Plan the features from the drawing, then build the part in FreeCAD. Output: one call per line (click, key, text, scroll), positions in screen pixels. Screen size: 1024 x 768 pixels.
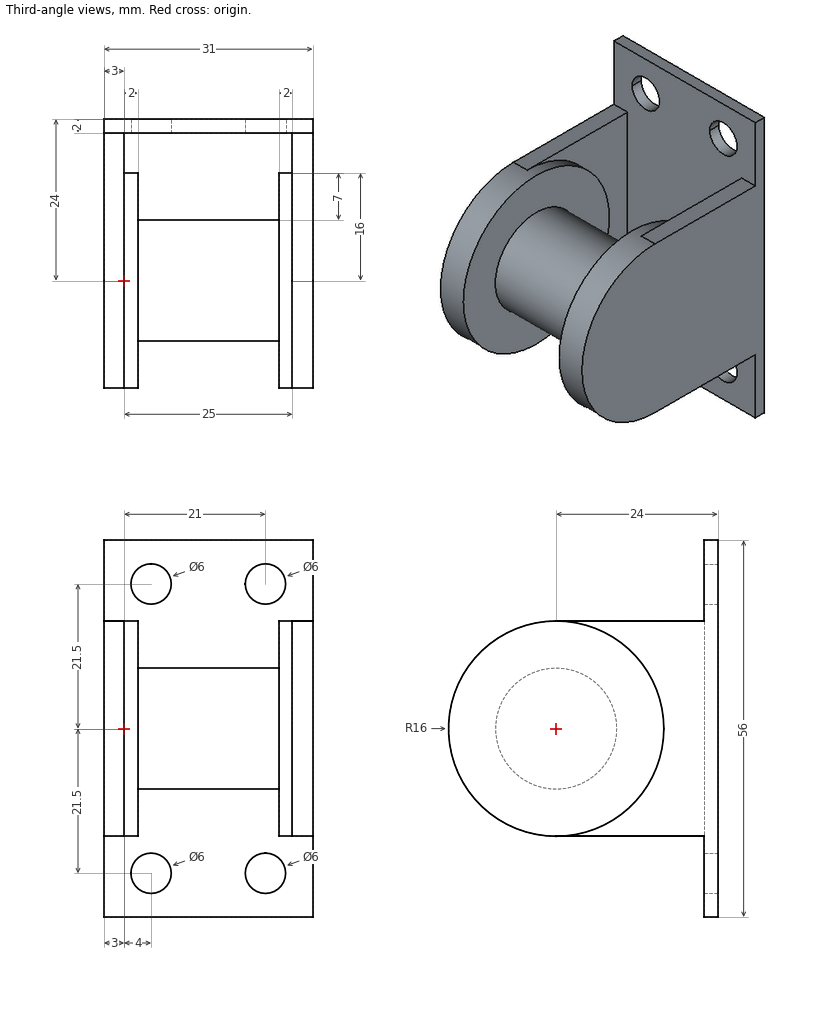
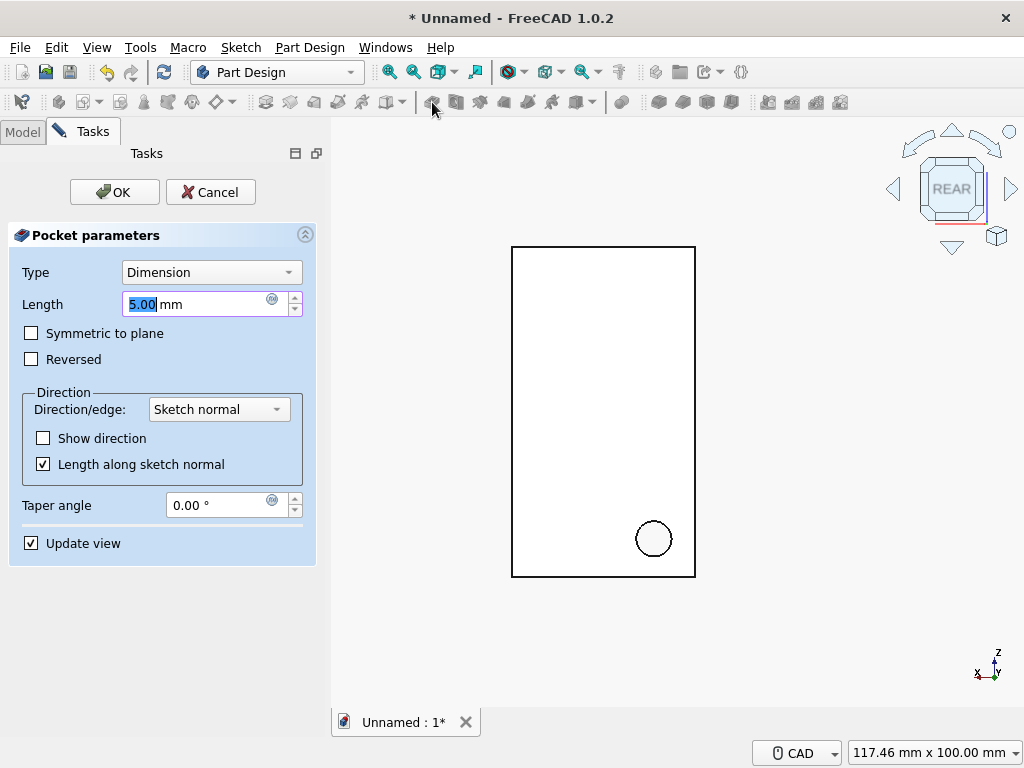
click(212, 272)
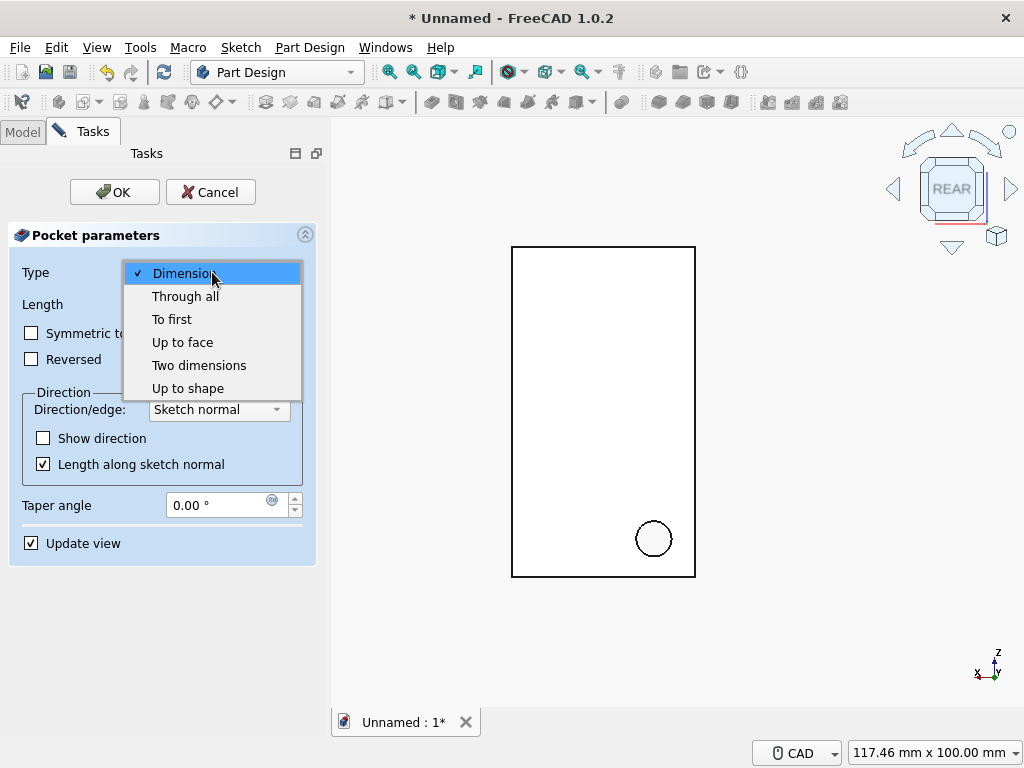
click(212, 320)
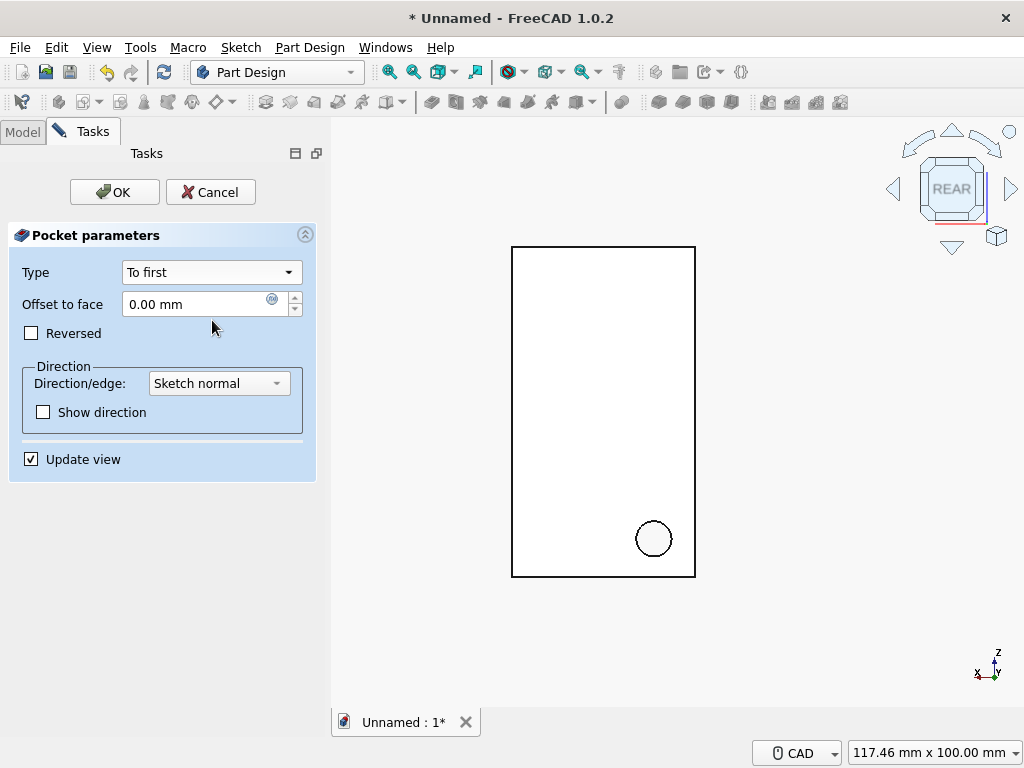
click(115, 192)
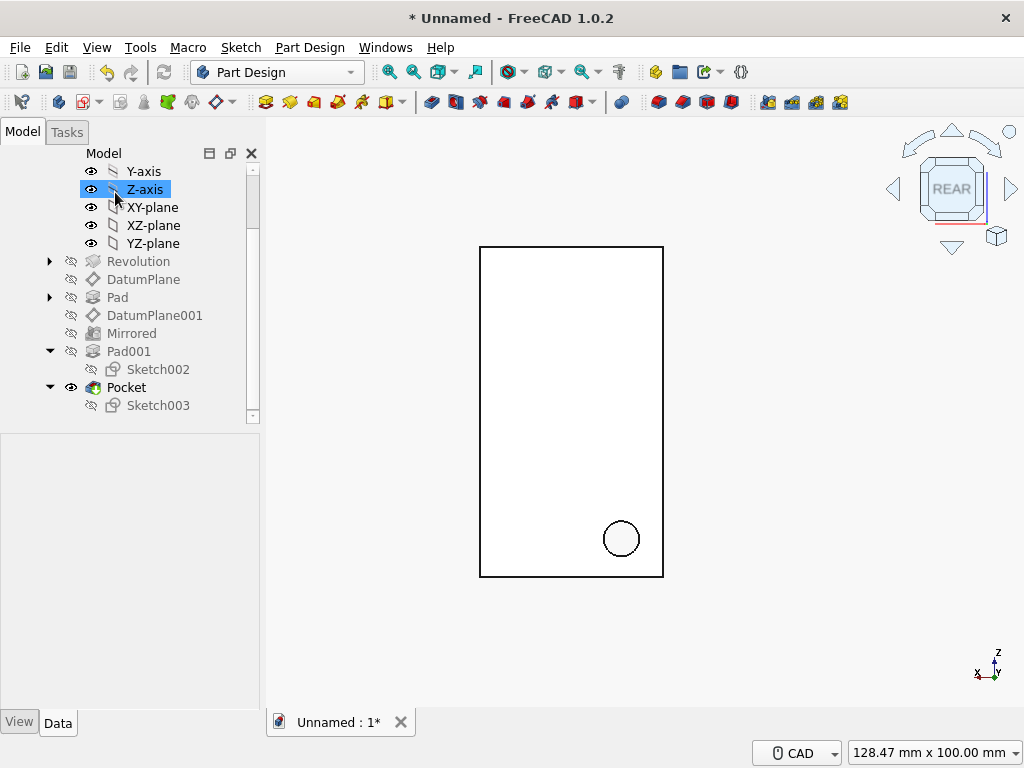
click(571, 364)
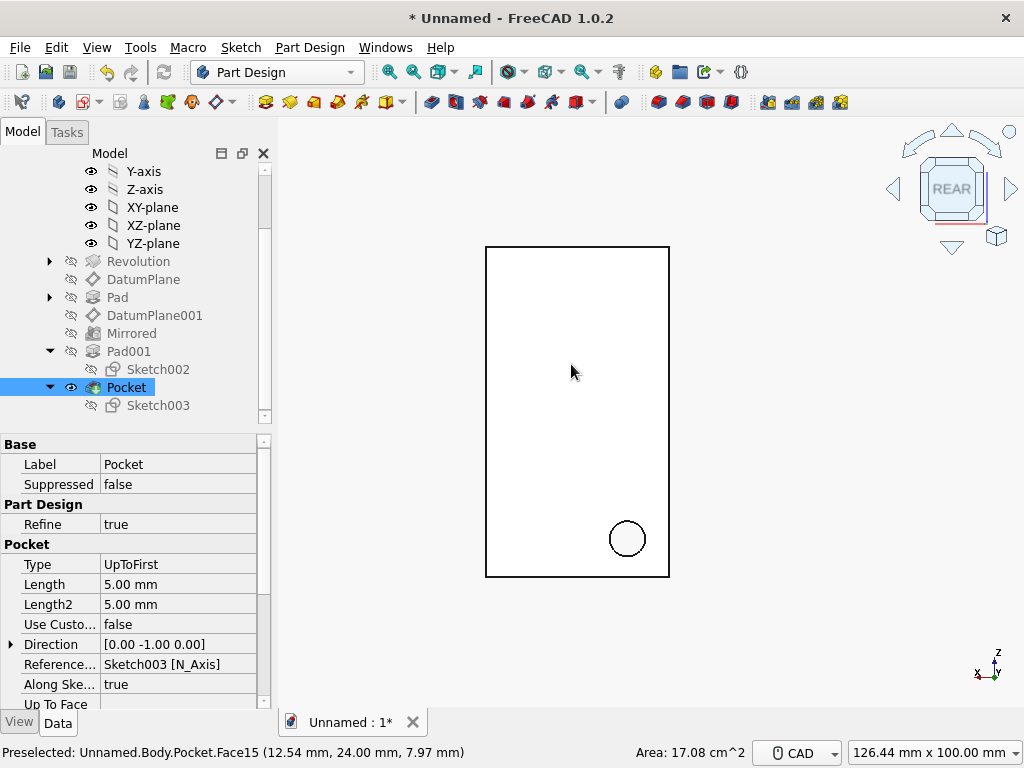
click(84, 102)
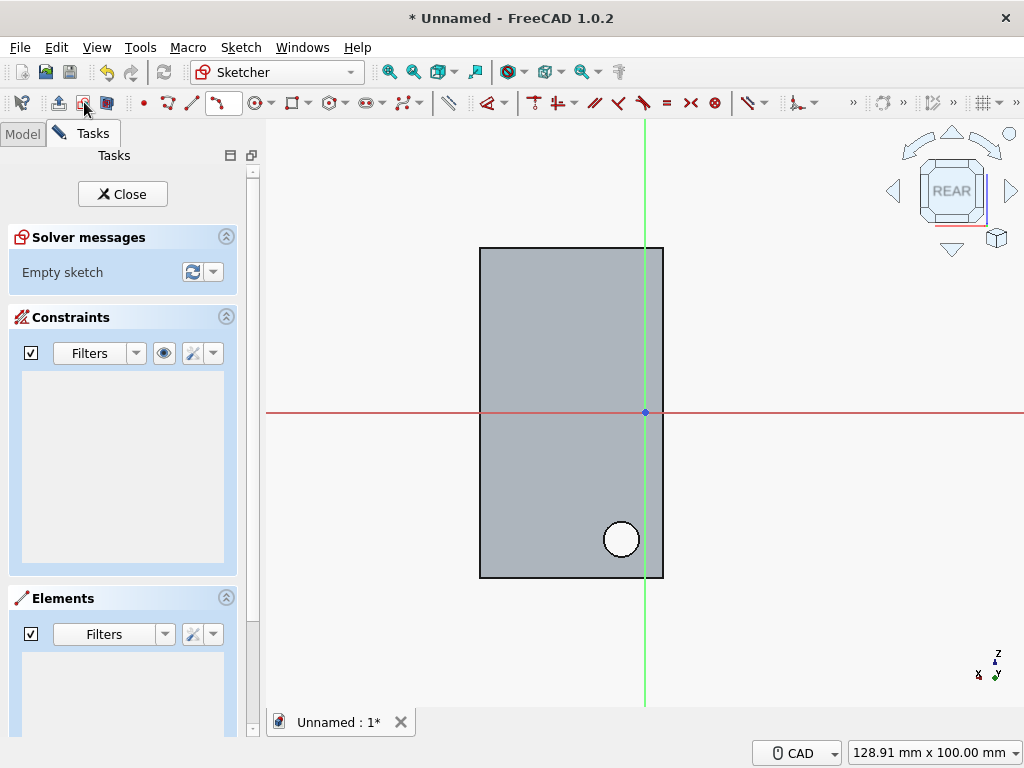
scroll(626, 274, up, 12)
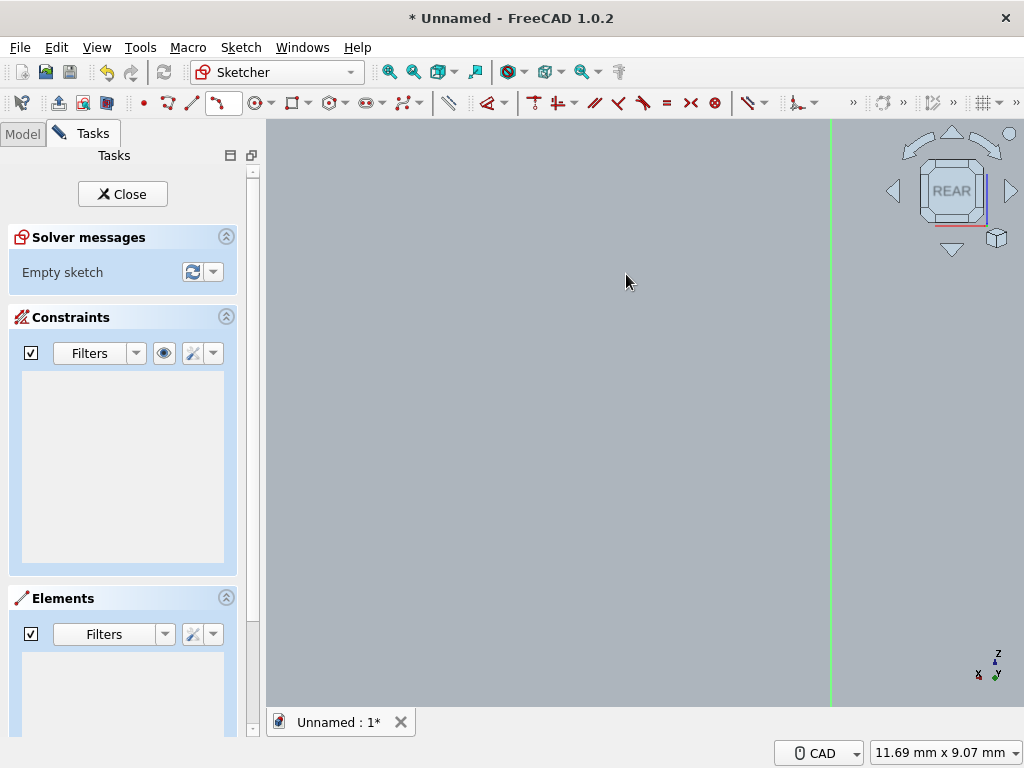
click(256, 104)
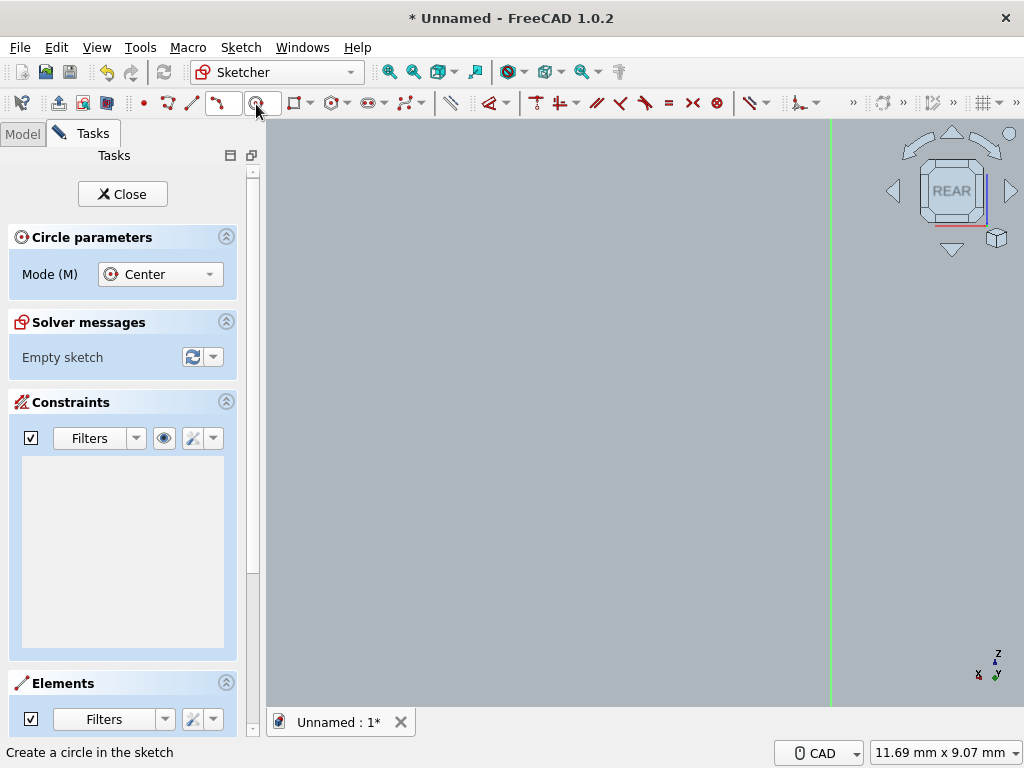
click(571, 410)
click(709, 273)
key(Escape)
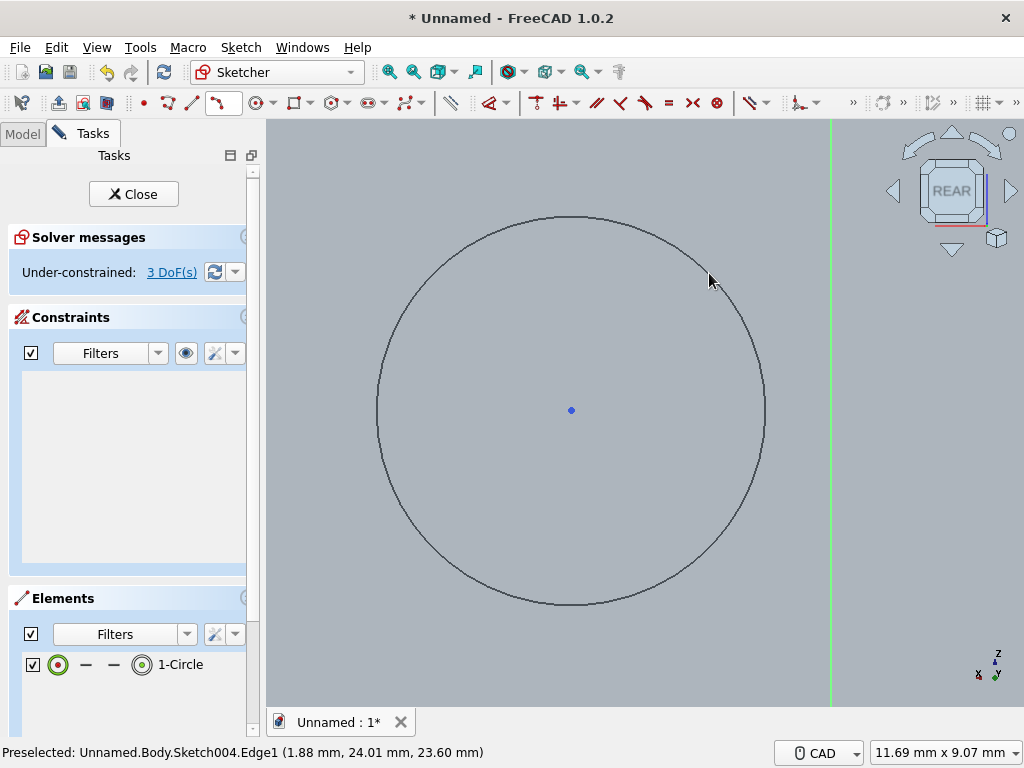
click(490, 104)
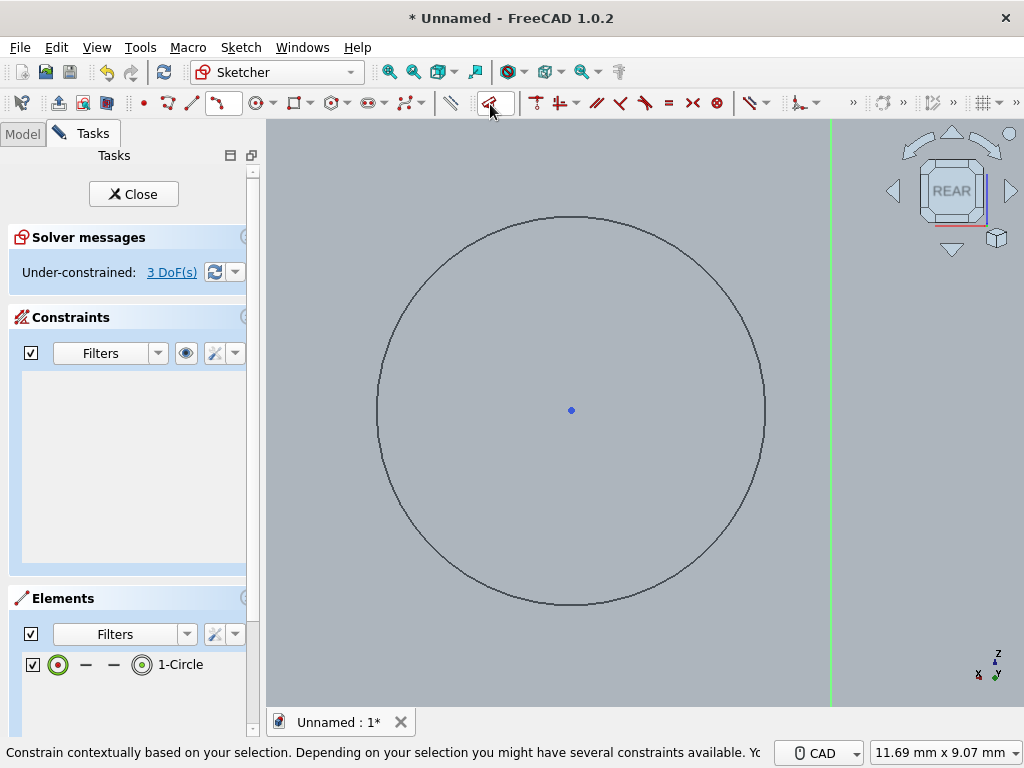
click(708, 273)
click(731, 250)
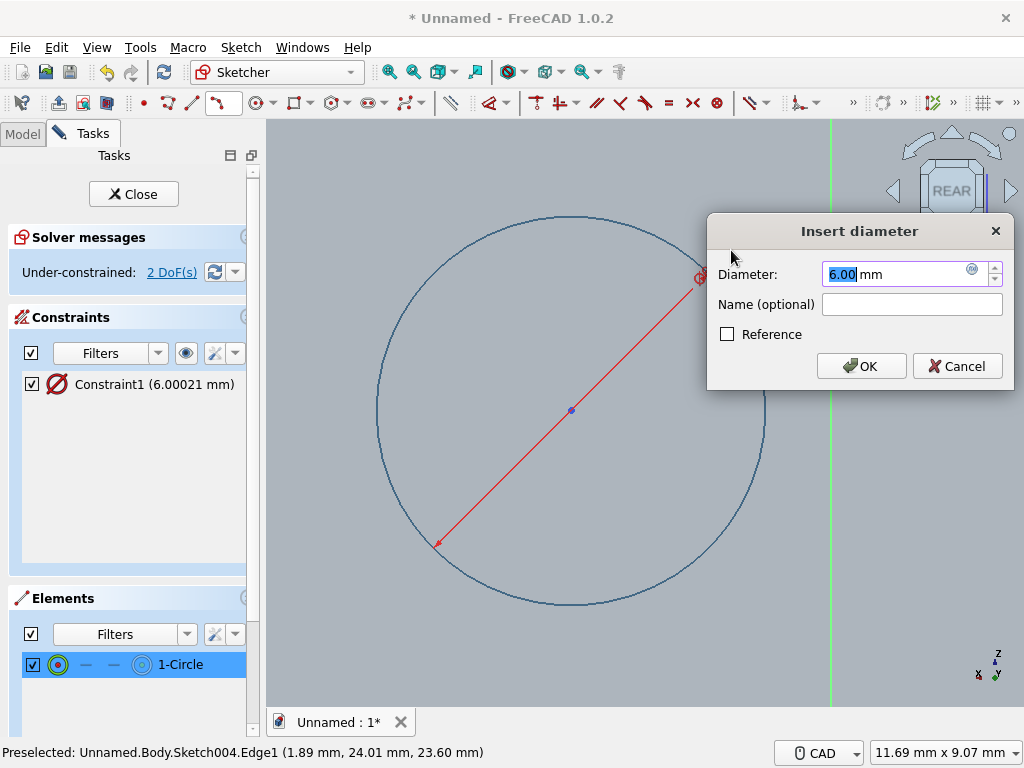
text(6)
key(Return)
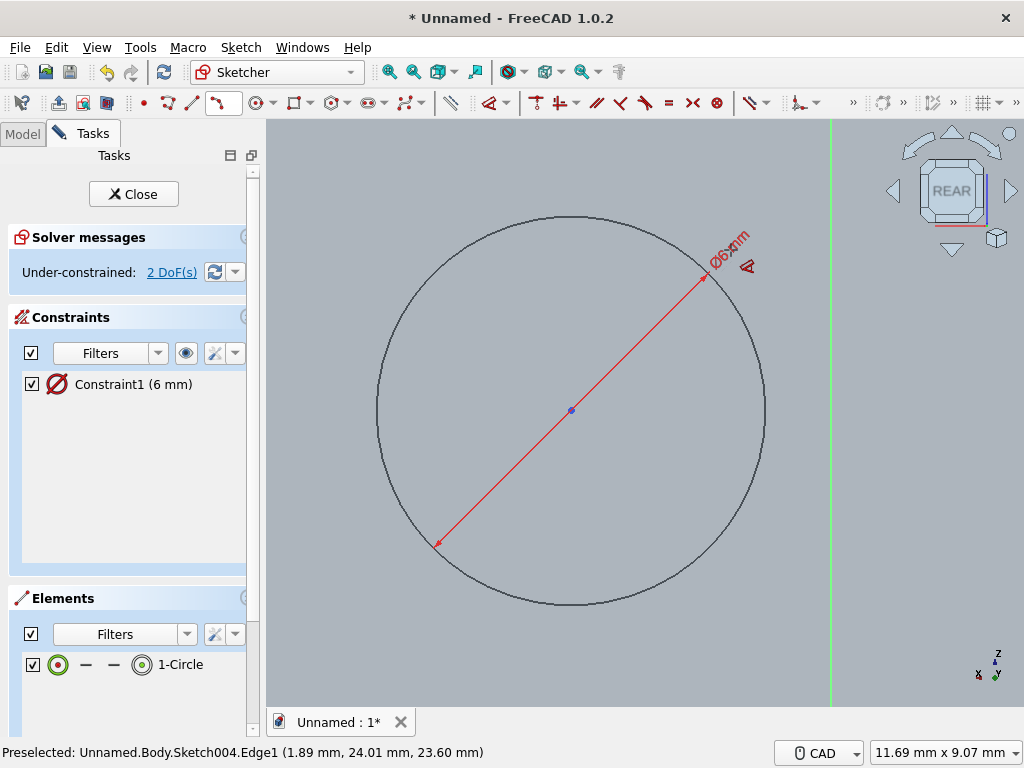
click(571, 411)
click(701, 377)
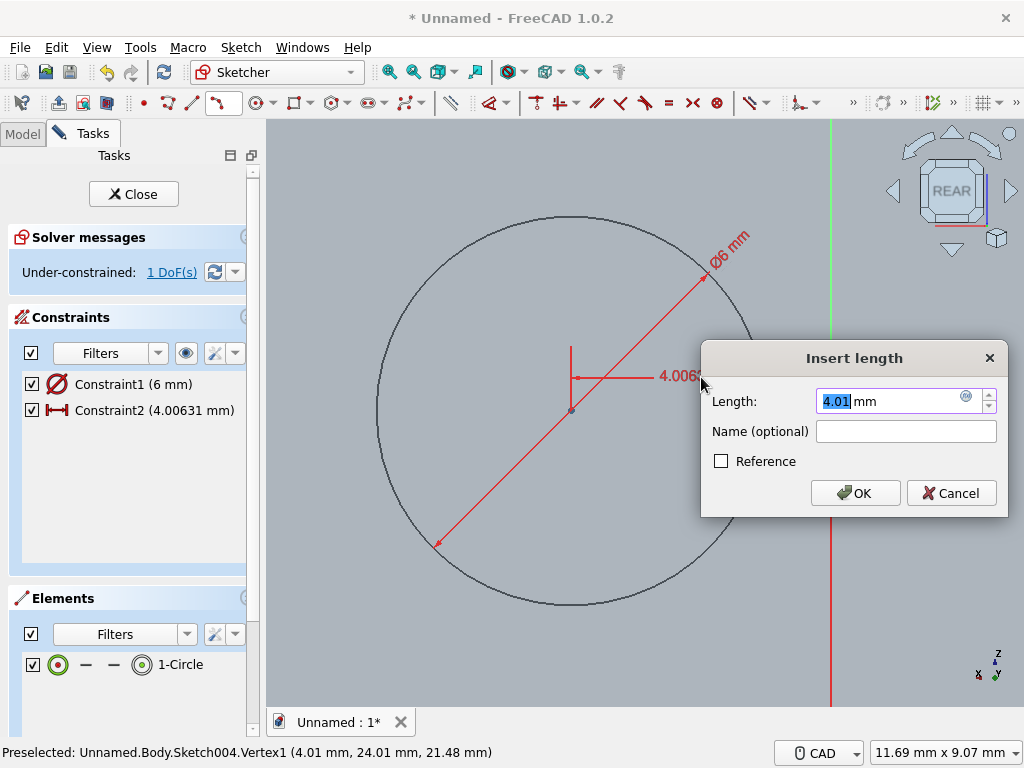
text(4)
key(Return)